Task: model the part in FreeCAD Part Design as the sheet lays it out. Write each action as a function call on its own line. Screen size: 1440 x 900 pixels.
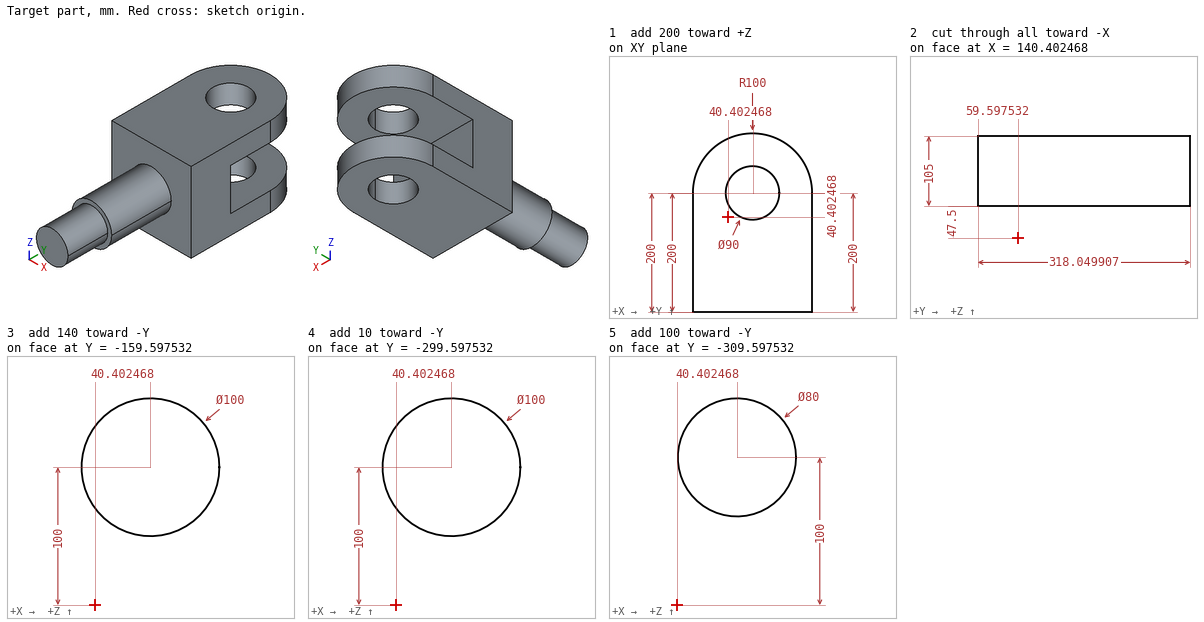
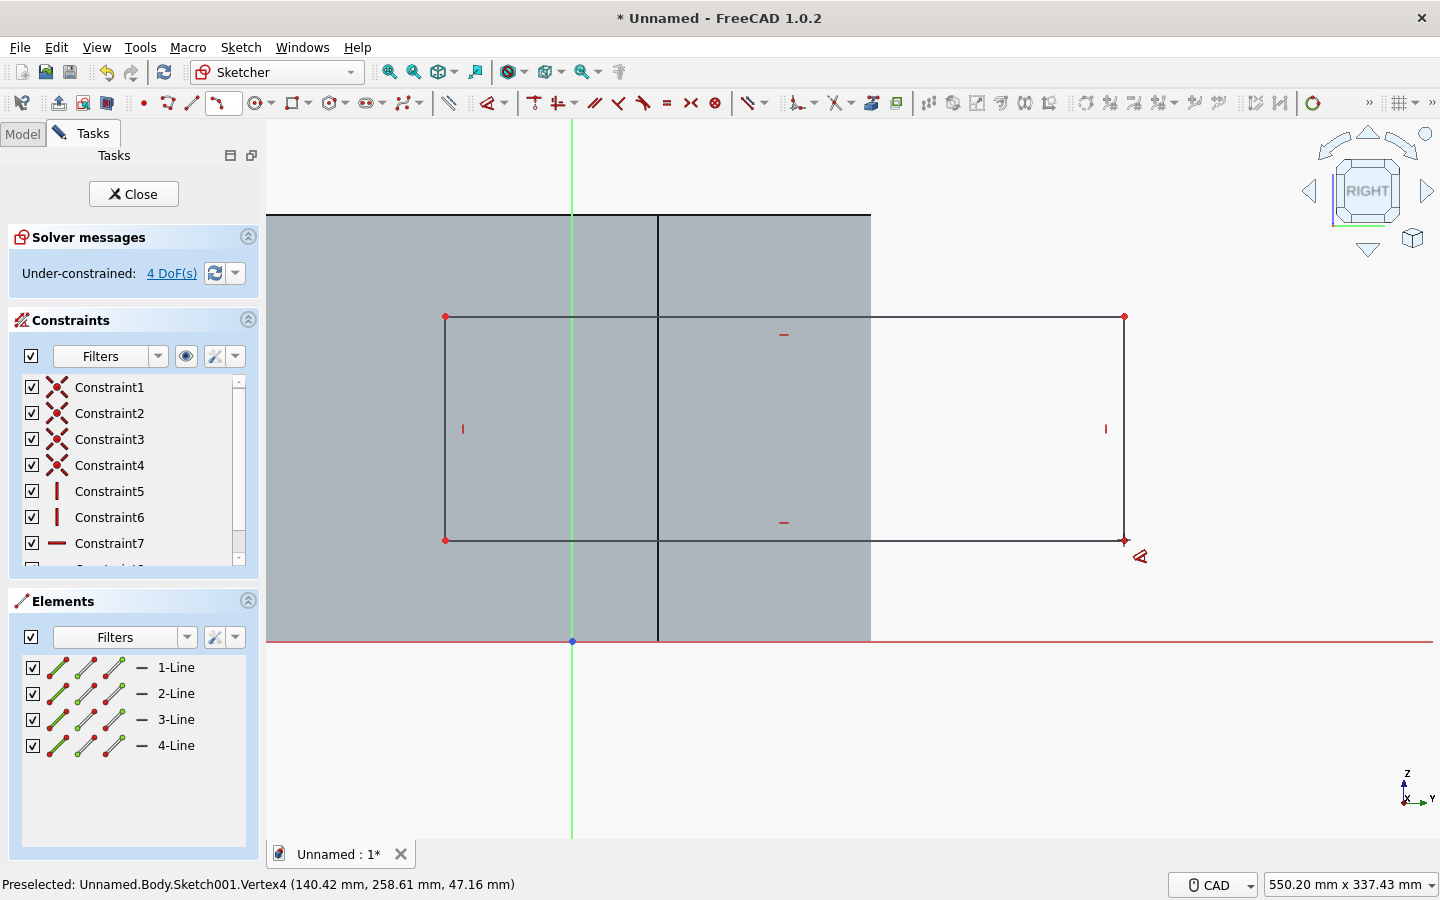
click(445, 384)
click(411, 429)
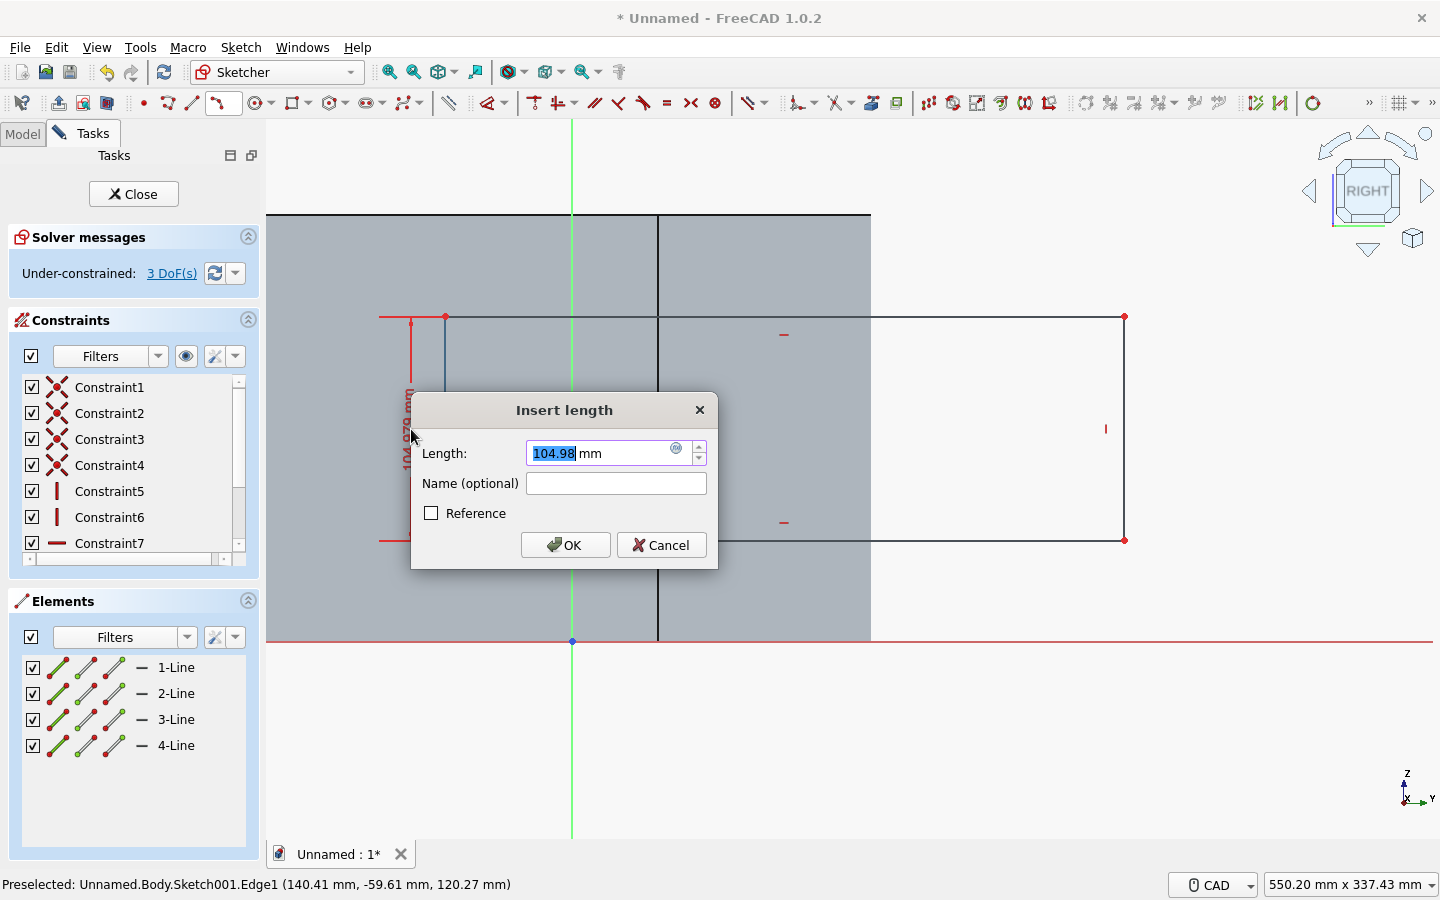
text(105)
key(Return)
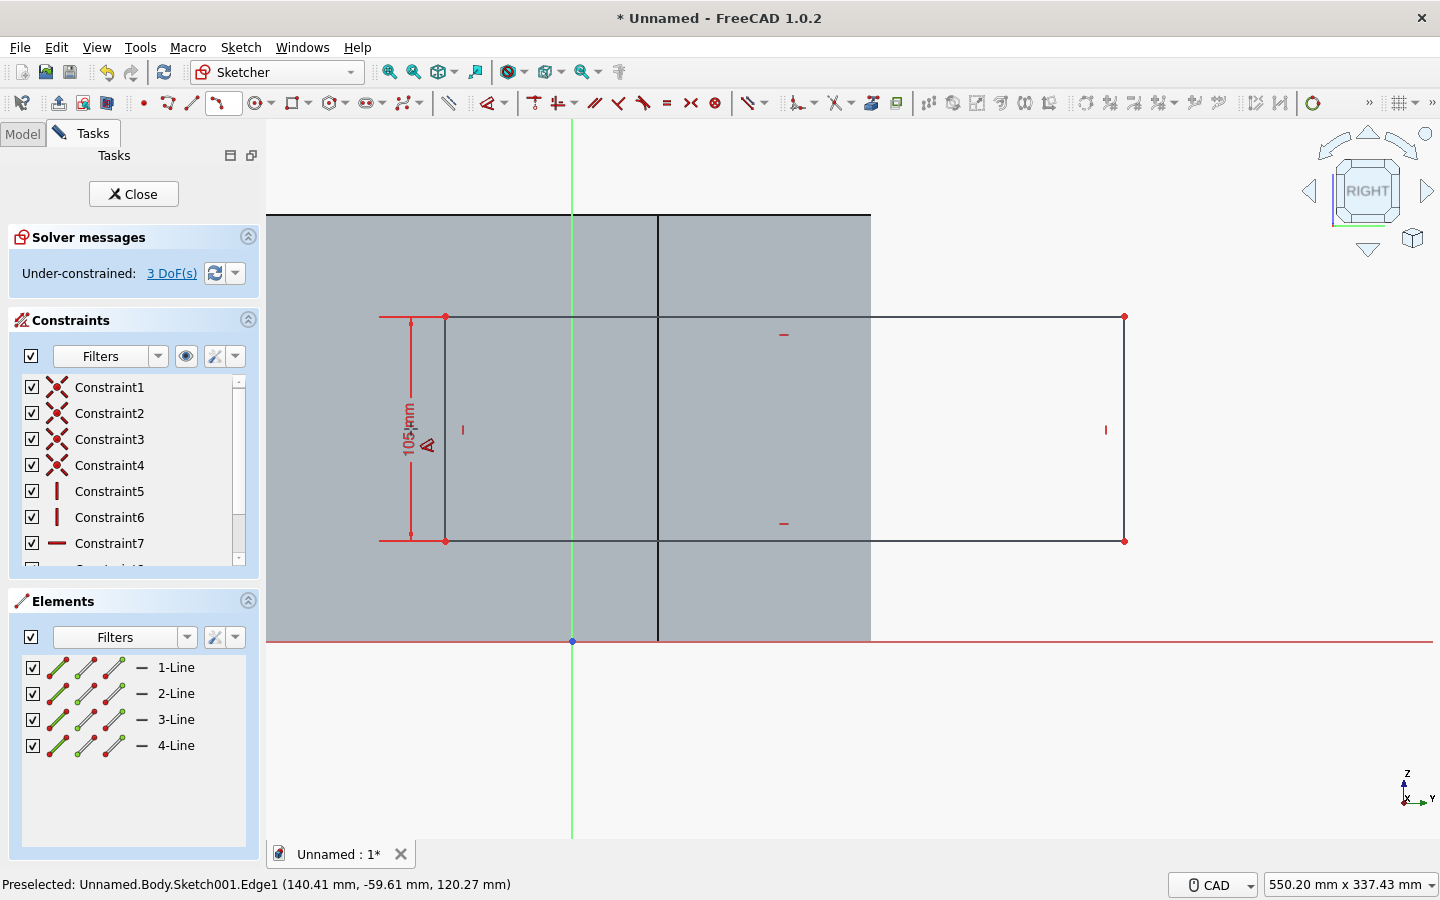
click(445, 541)
click(411, 591)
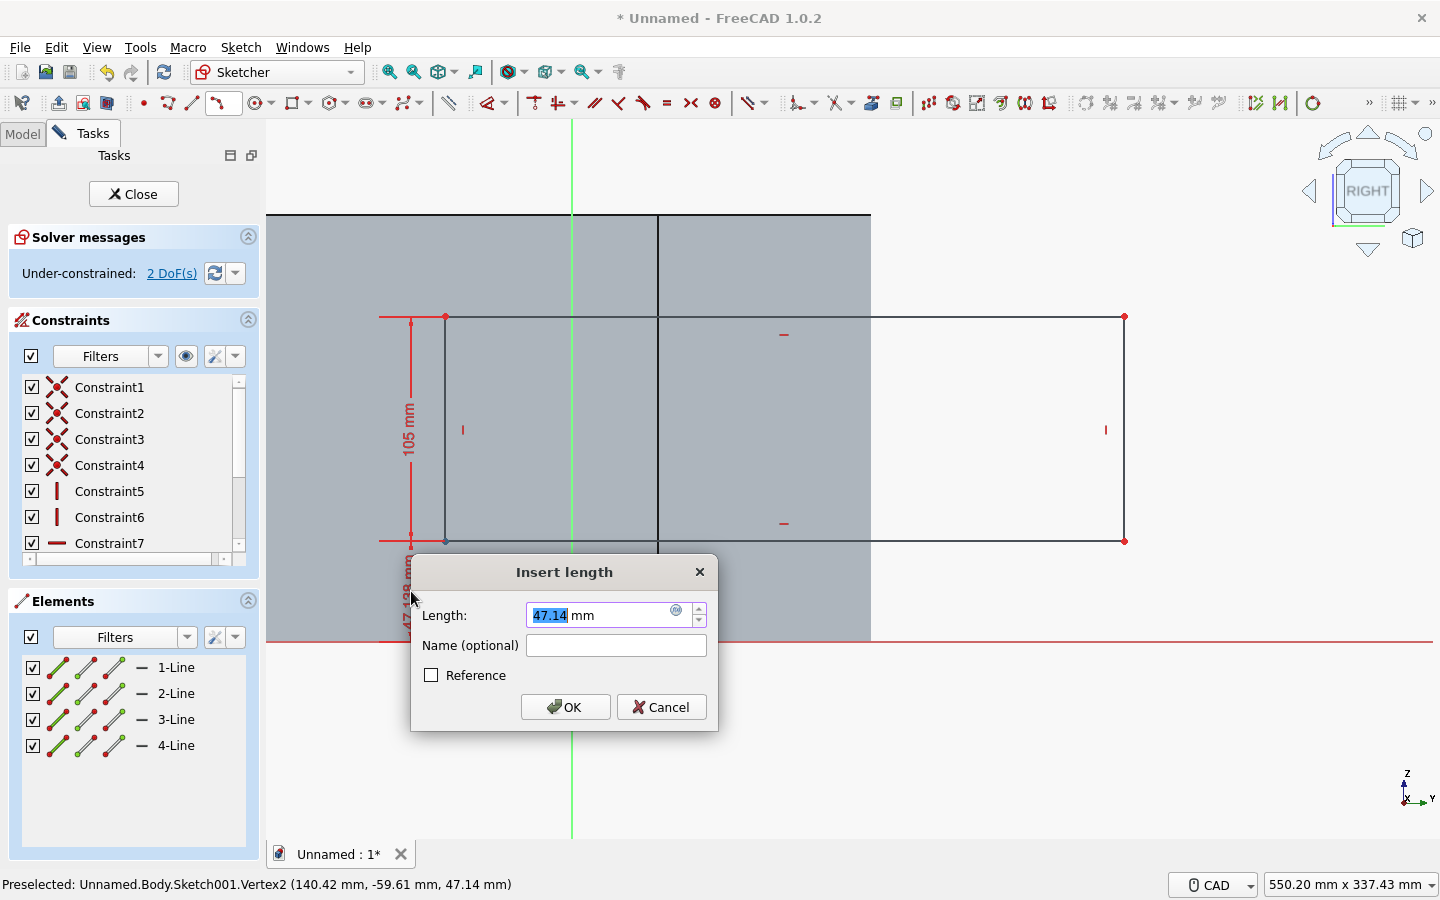
text(47.5)
key(Return)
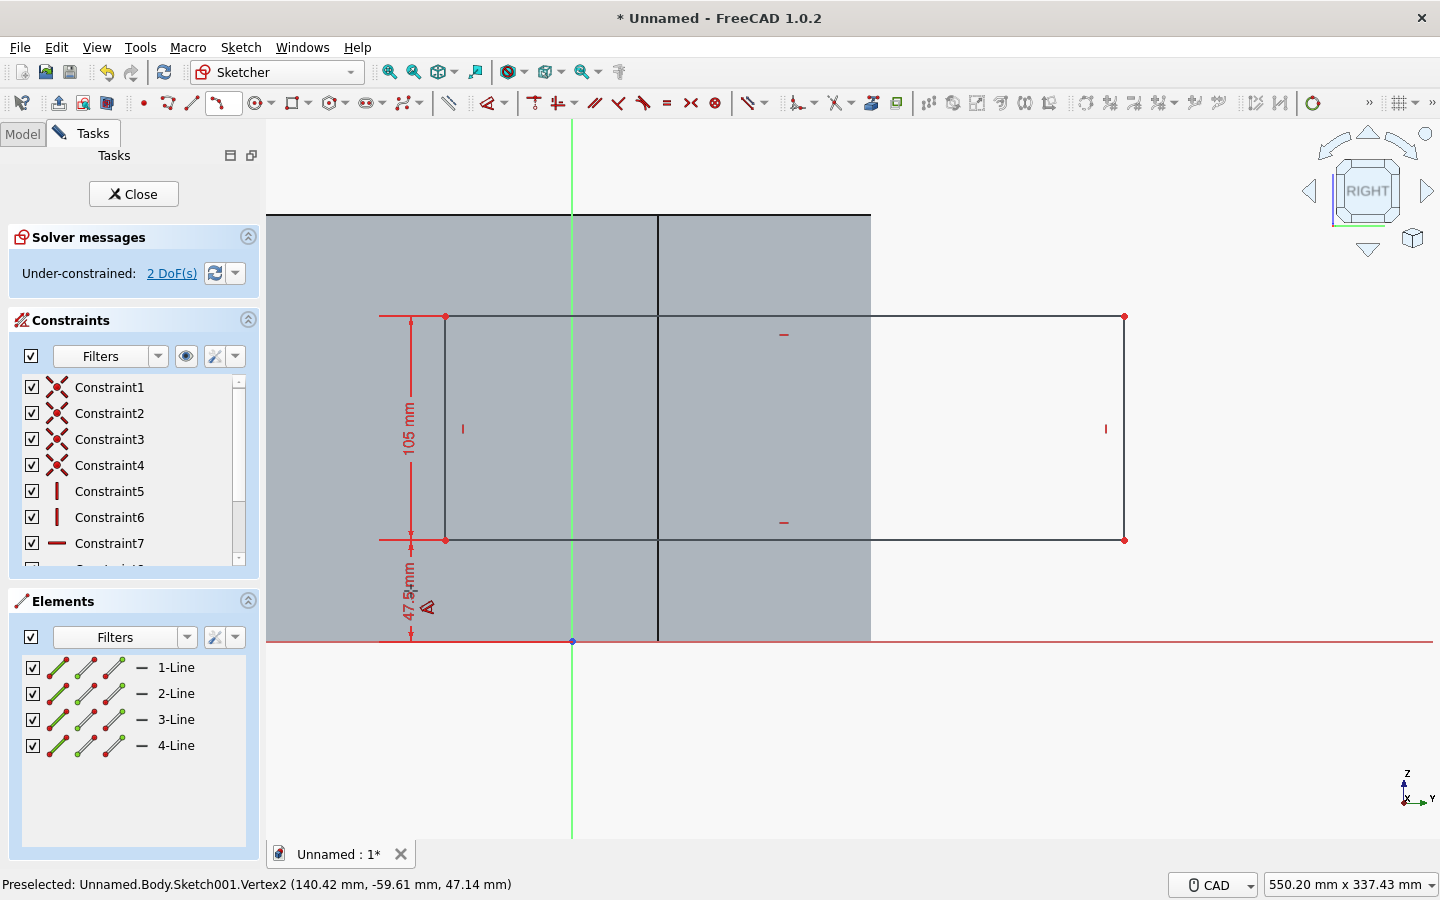
click(649, 540)
click(785, 574)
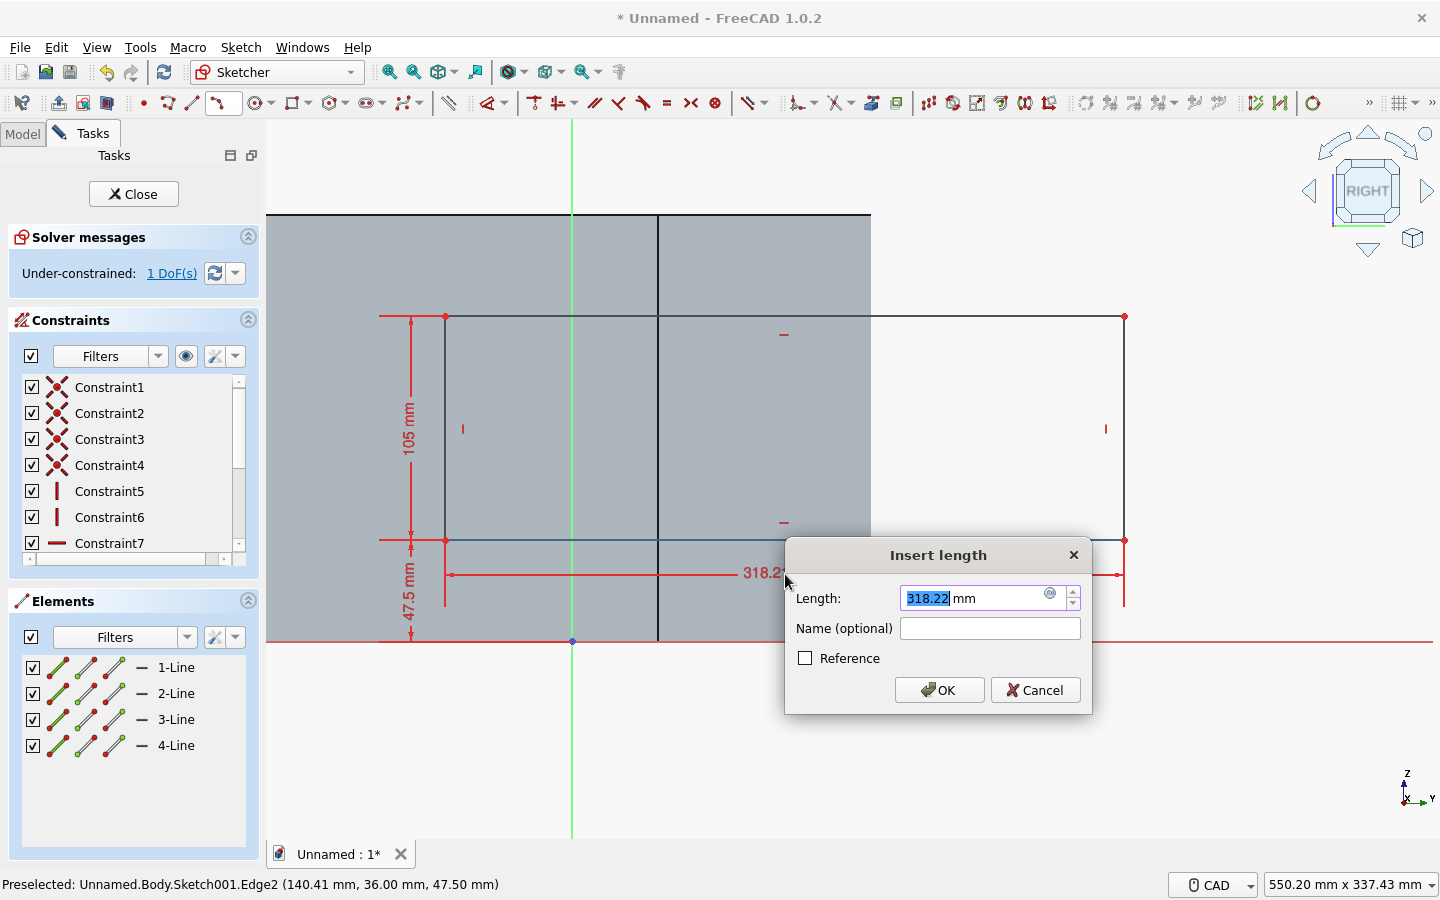
text(318.049907)
key(Return)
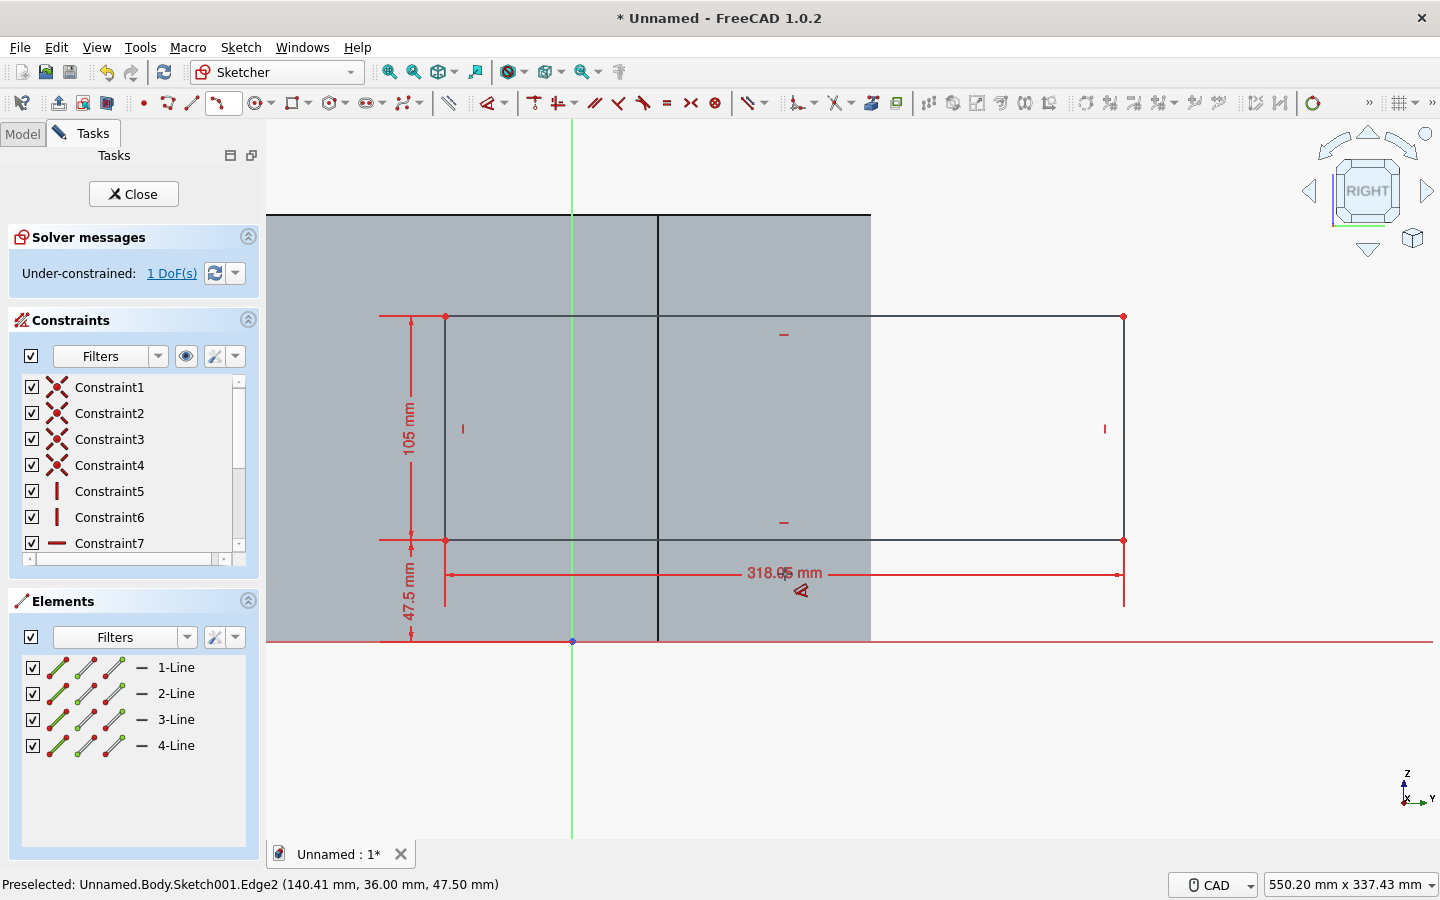
click(445, 316)
click(509, 676)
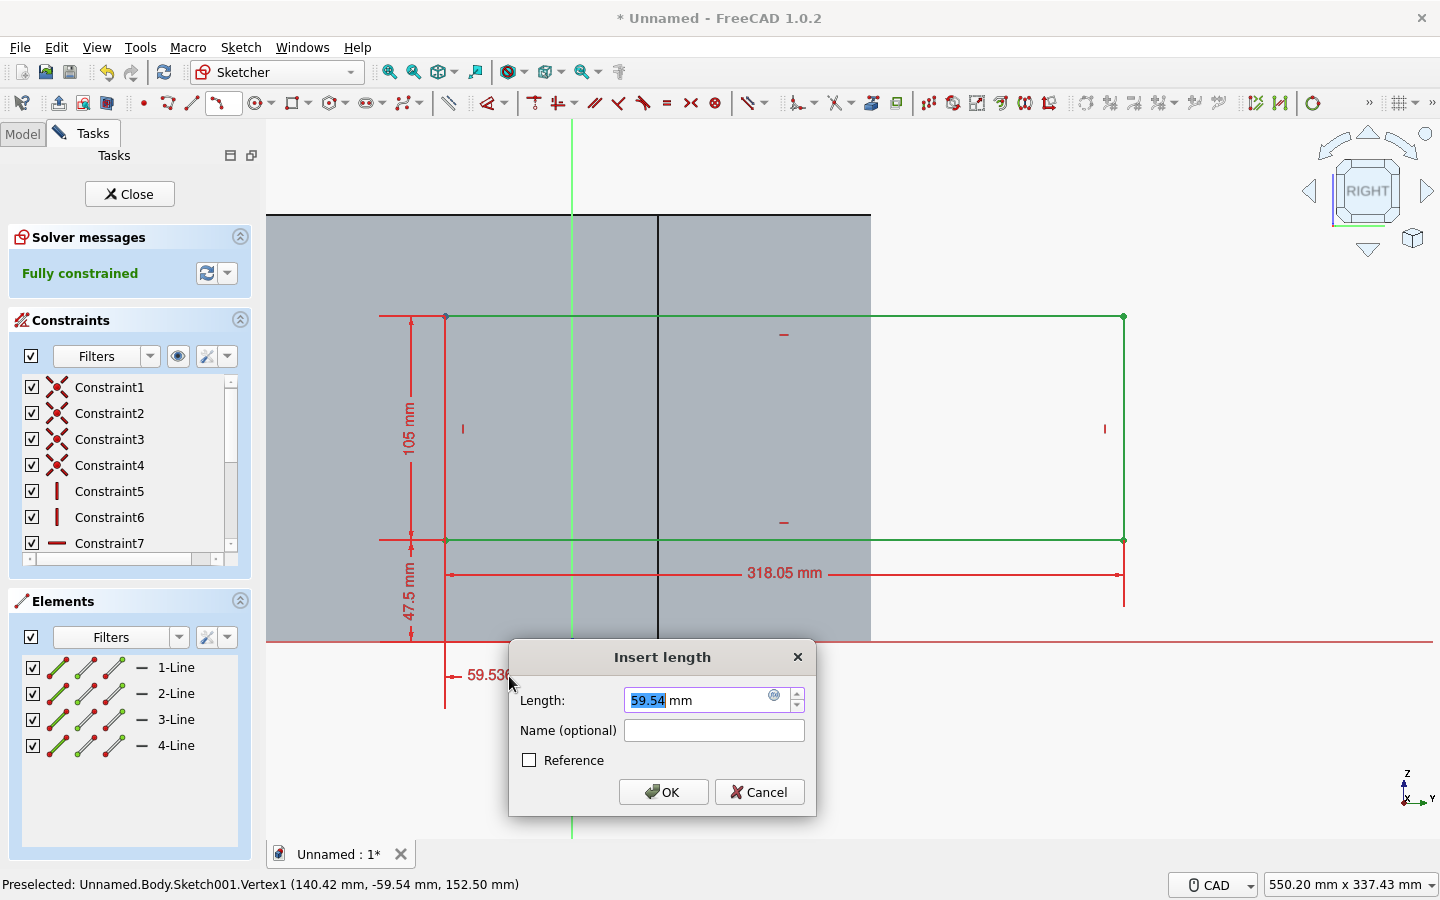
text(59.597532)
key(Return)
key(Escape)